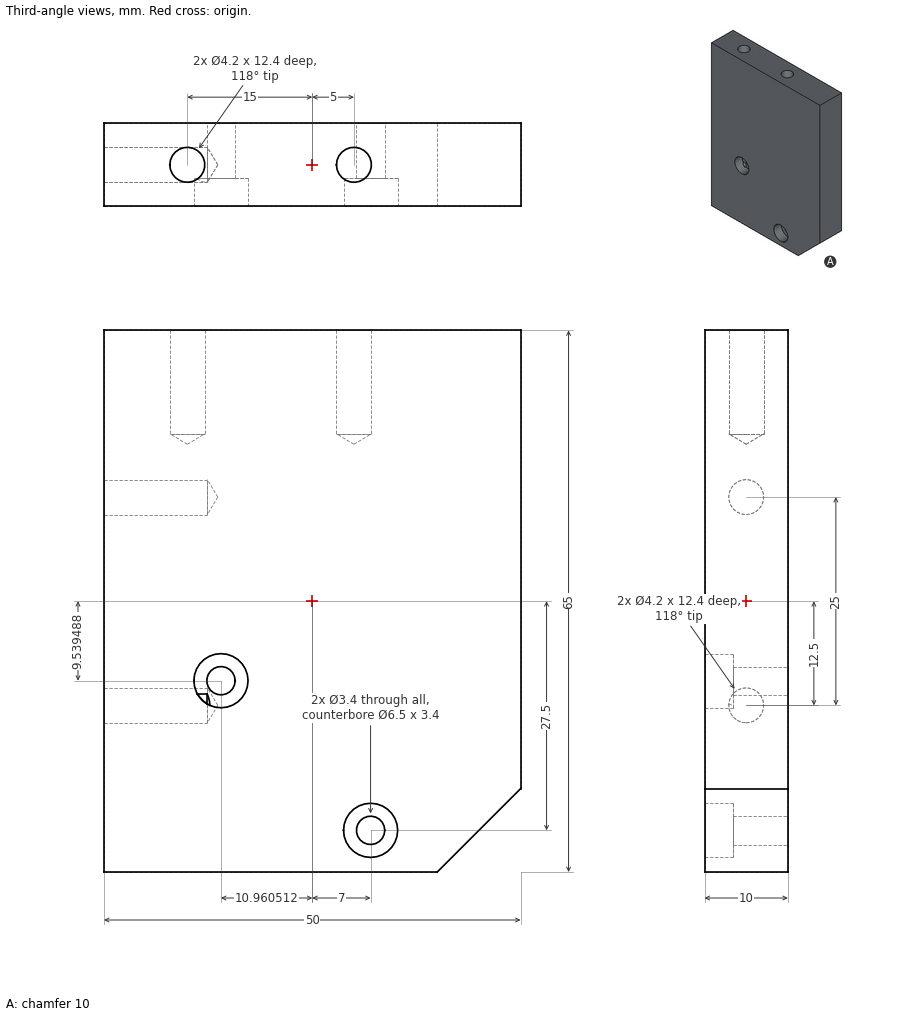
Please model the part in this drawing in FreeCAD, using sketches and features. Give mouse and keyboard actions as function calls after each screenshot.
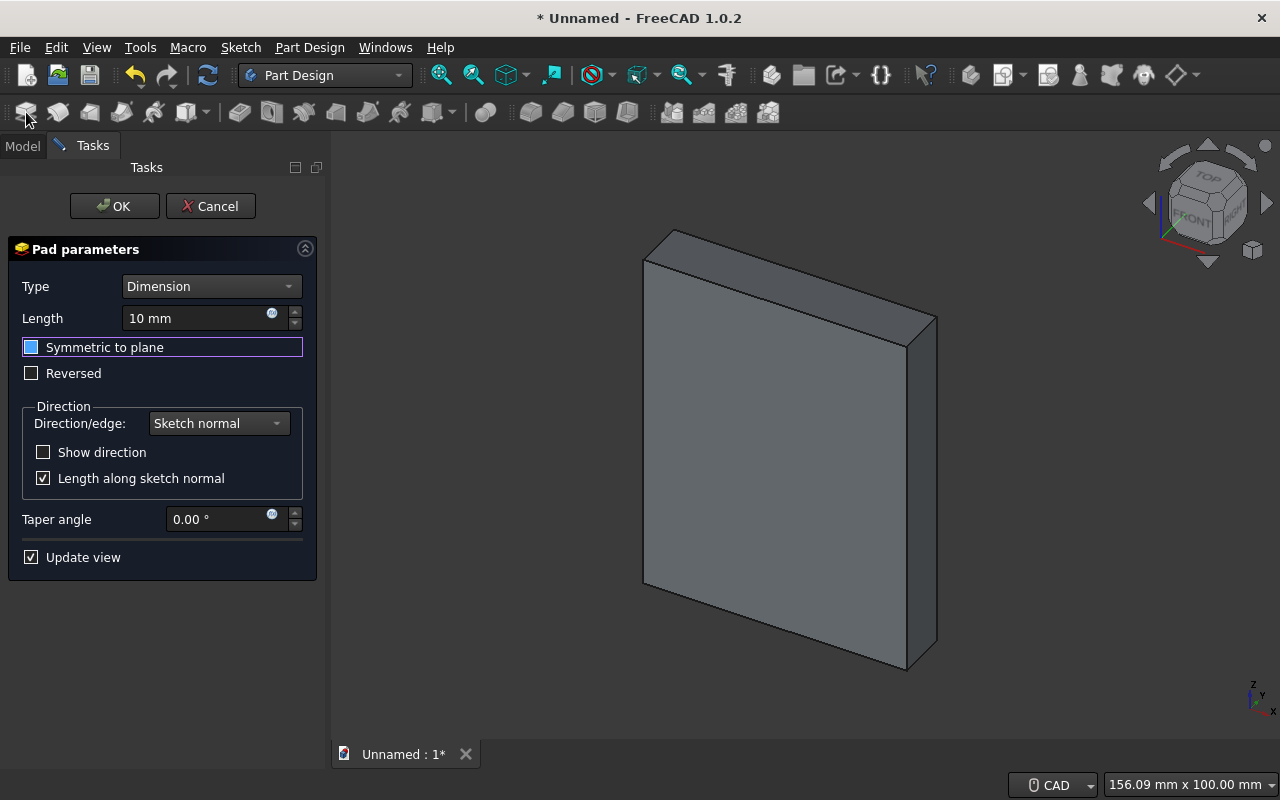
click(30, 347)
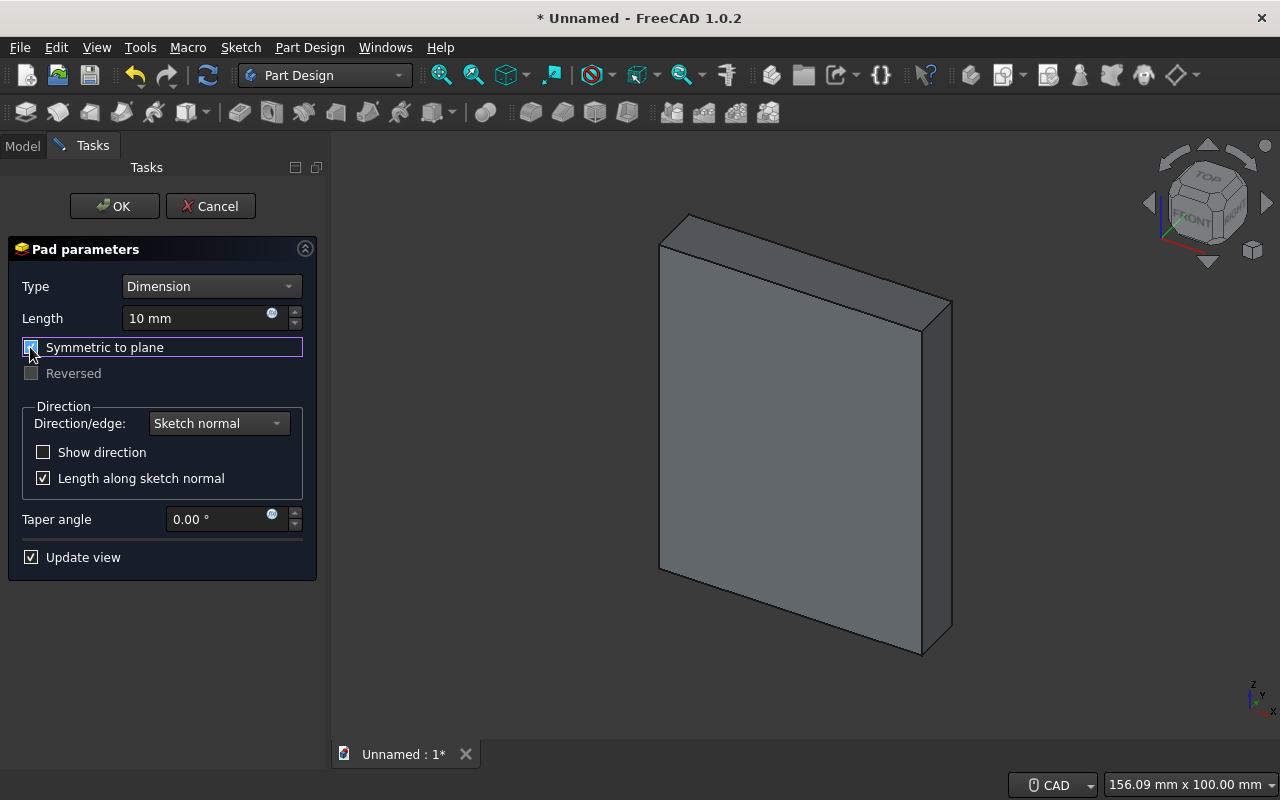
click(115, 206)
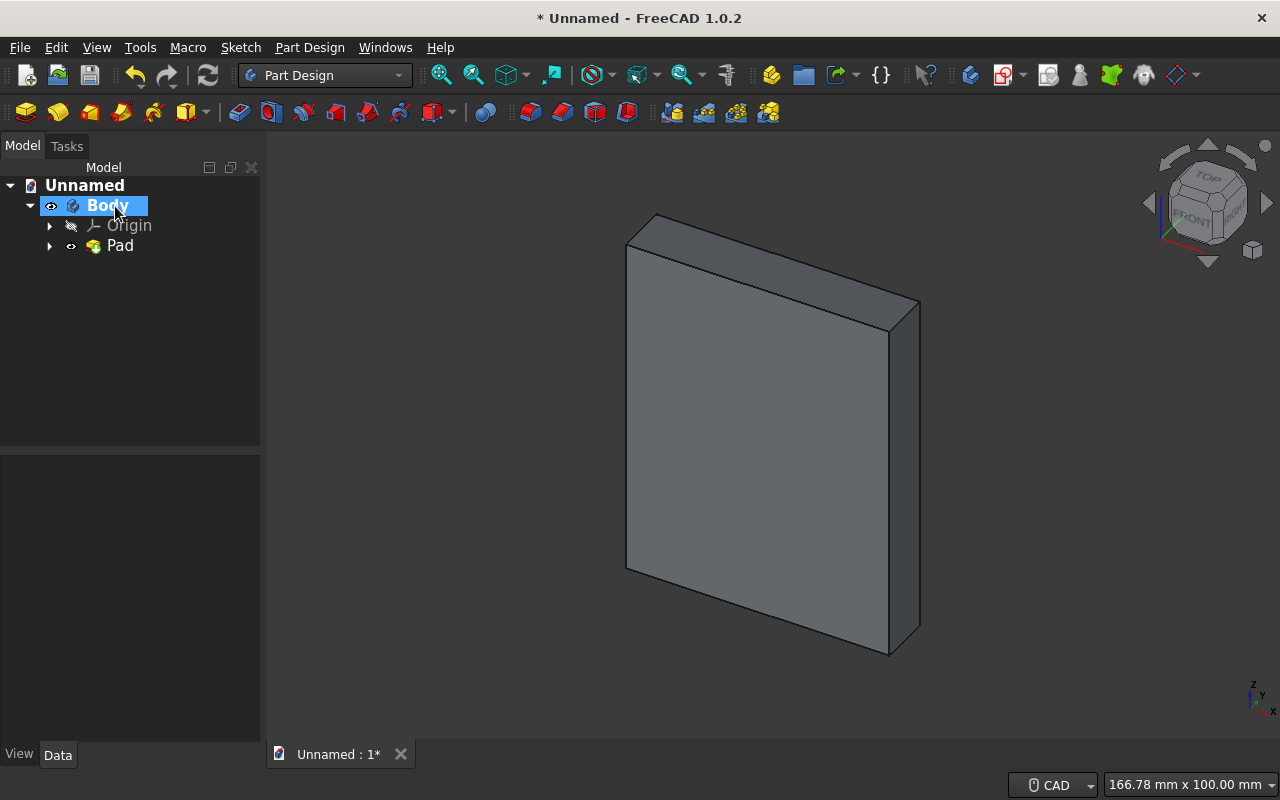
key(0)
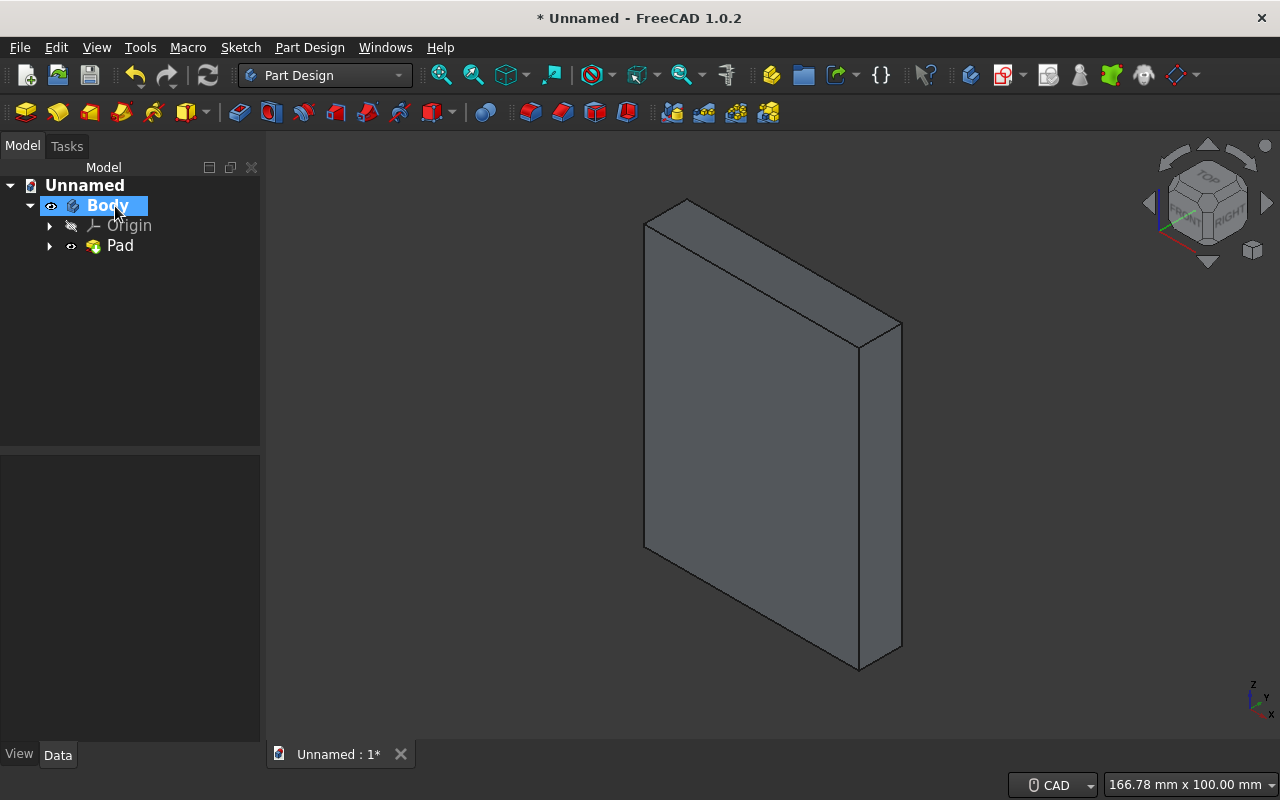
key(2)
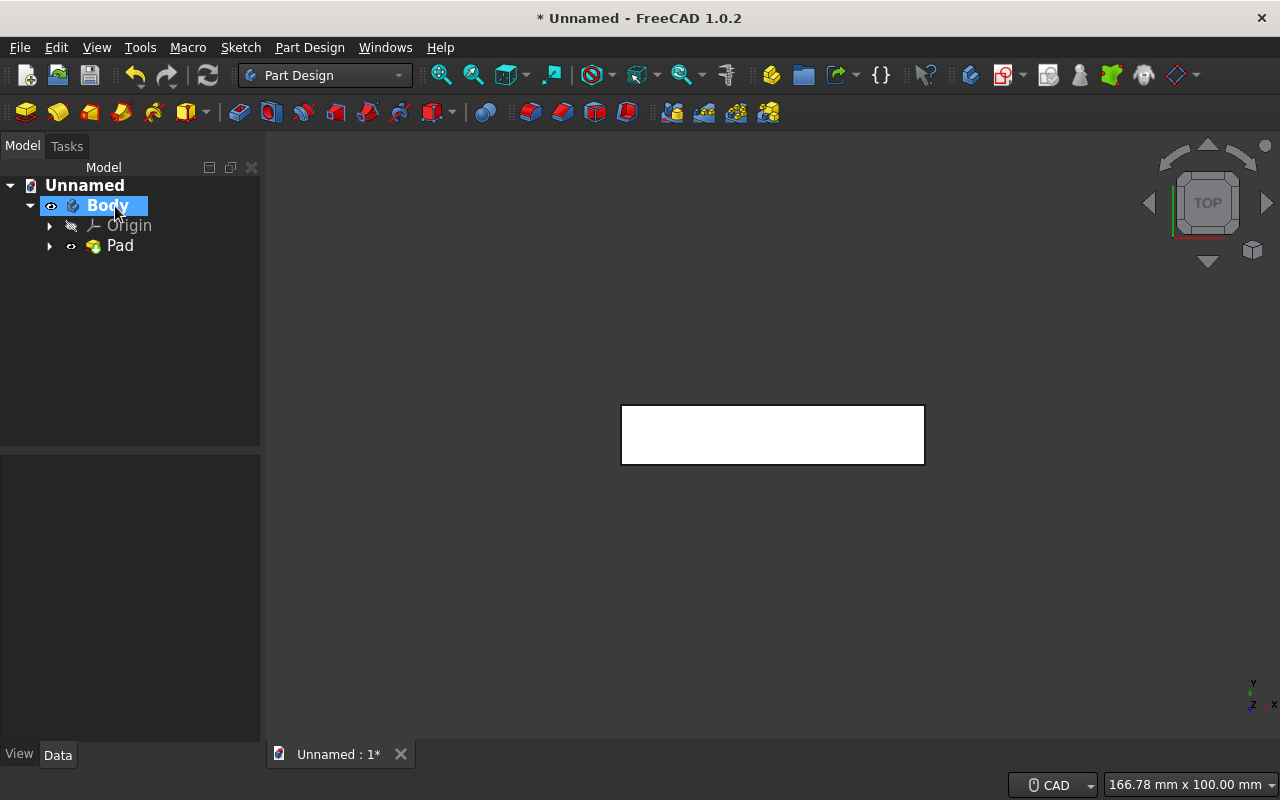
key(v)
key(f)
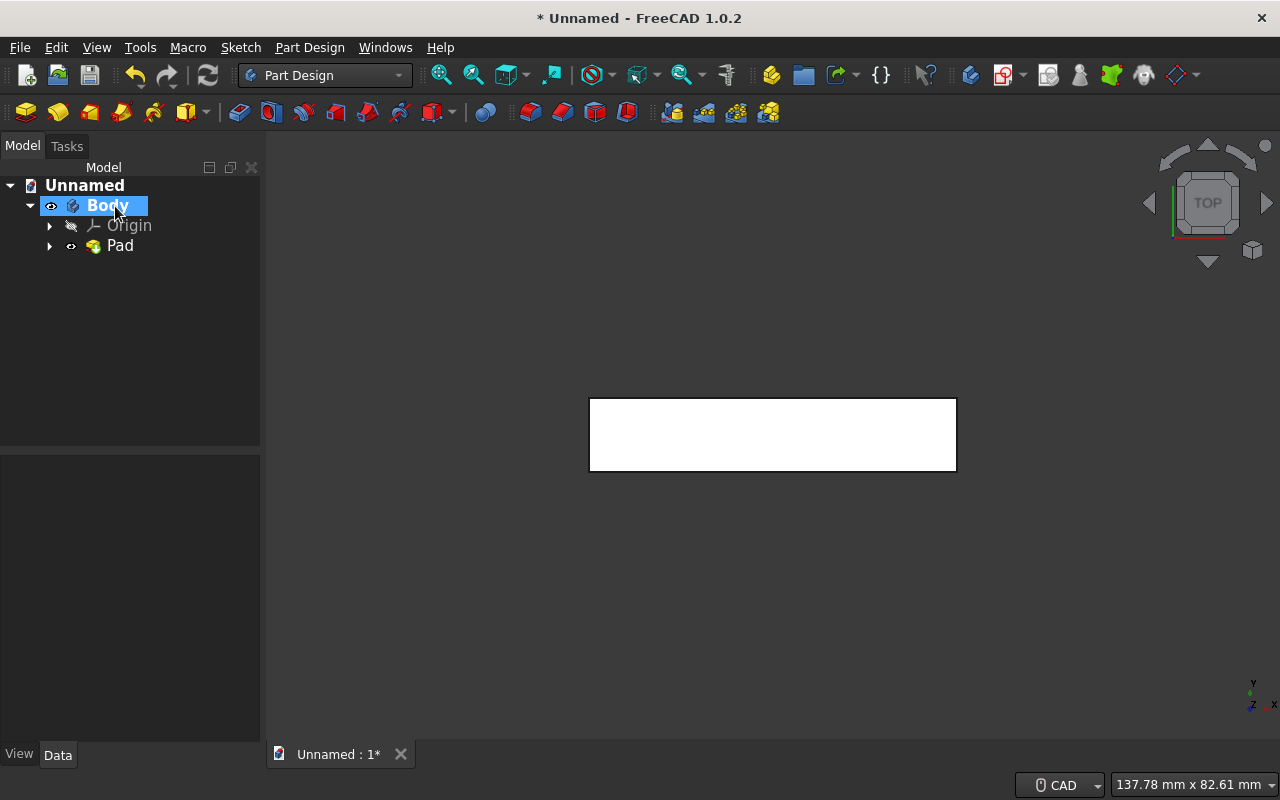
key(1)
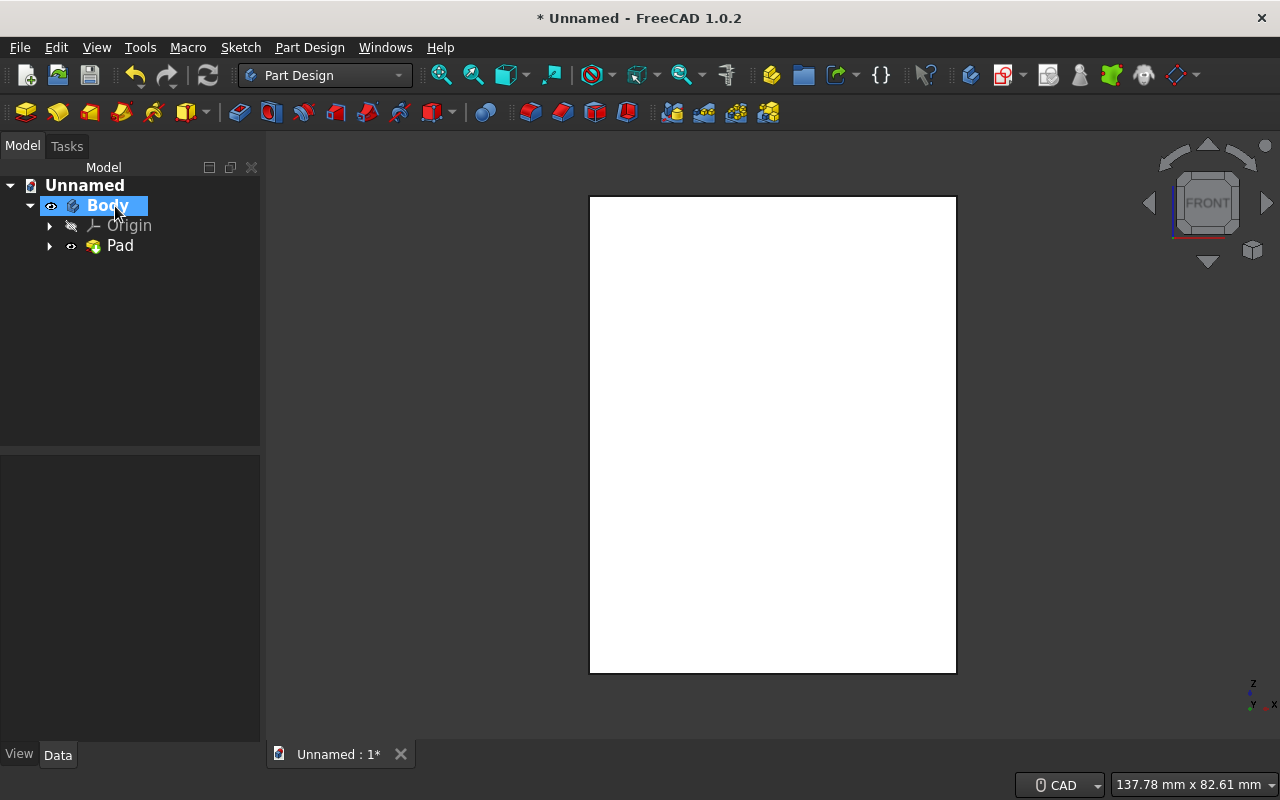
key(3)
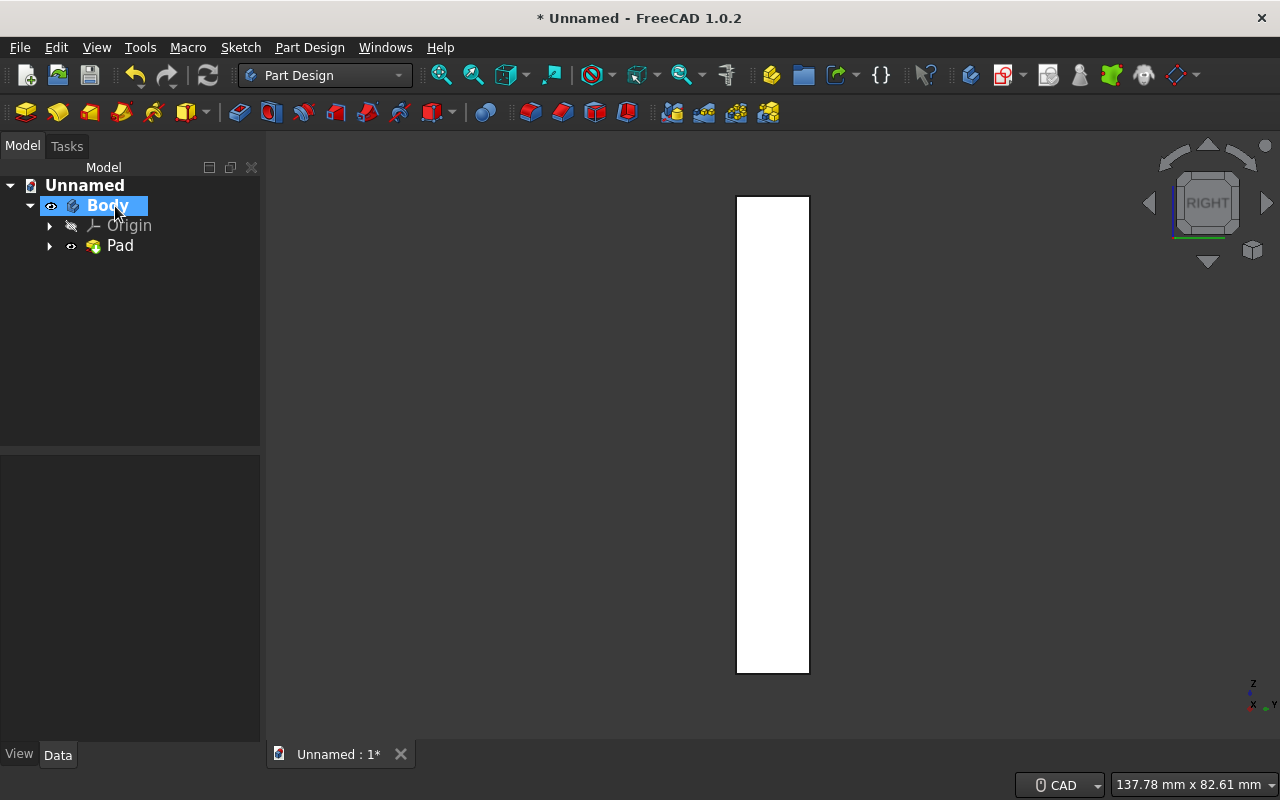
click(773, 673)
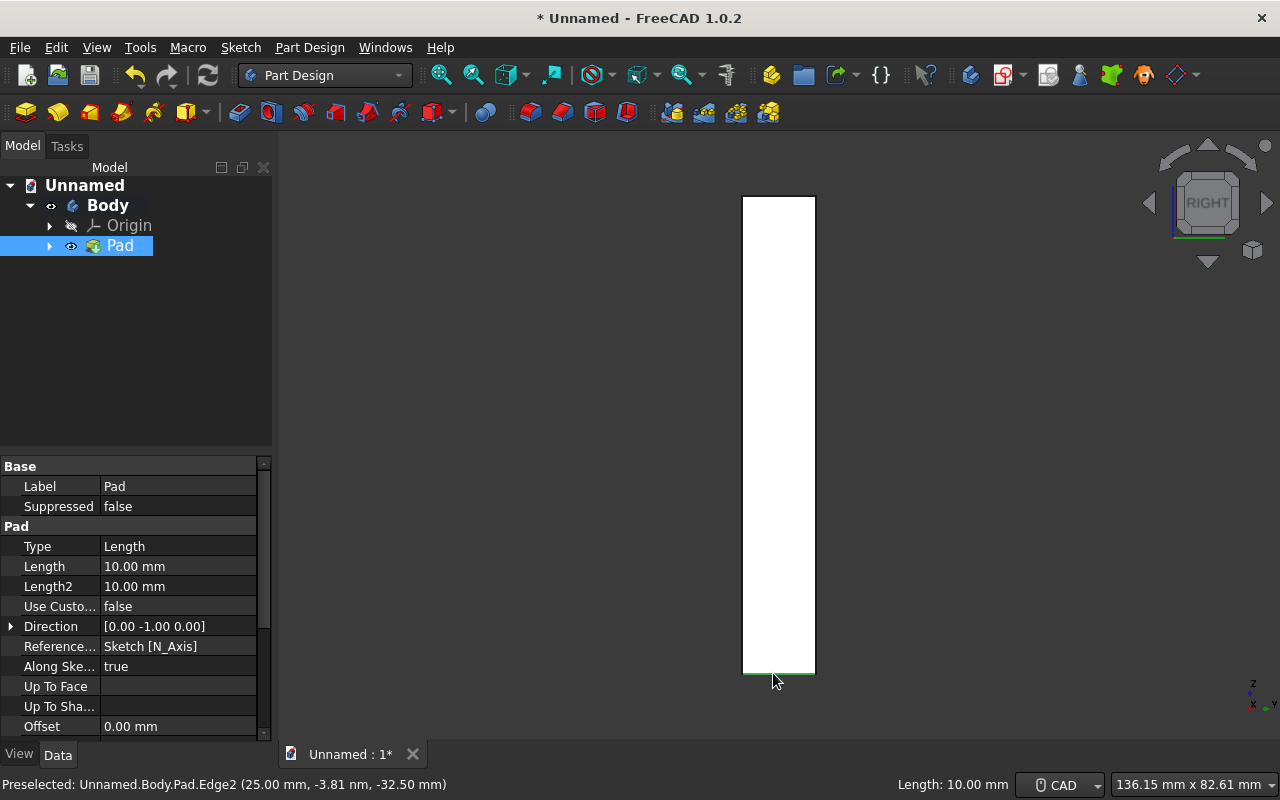
click(564, 112)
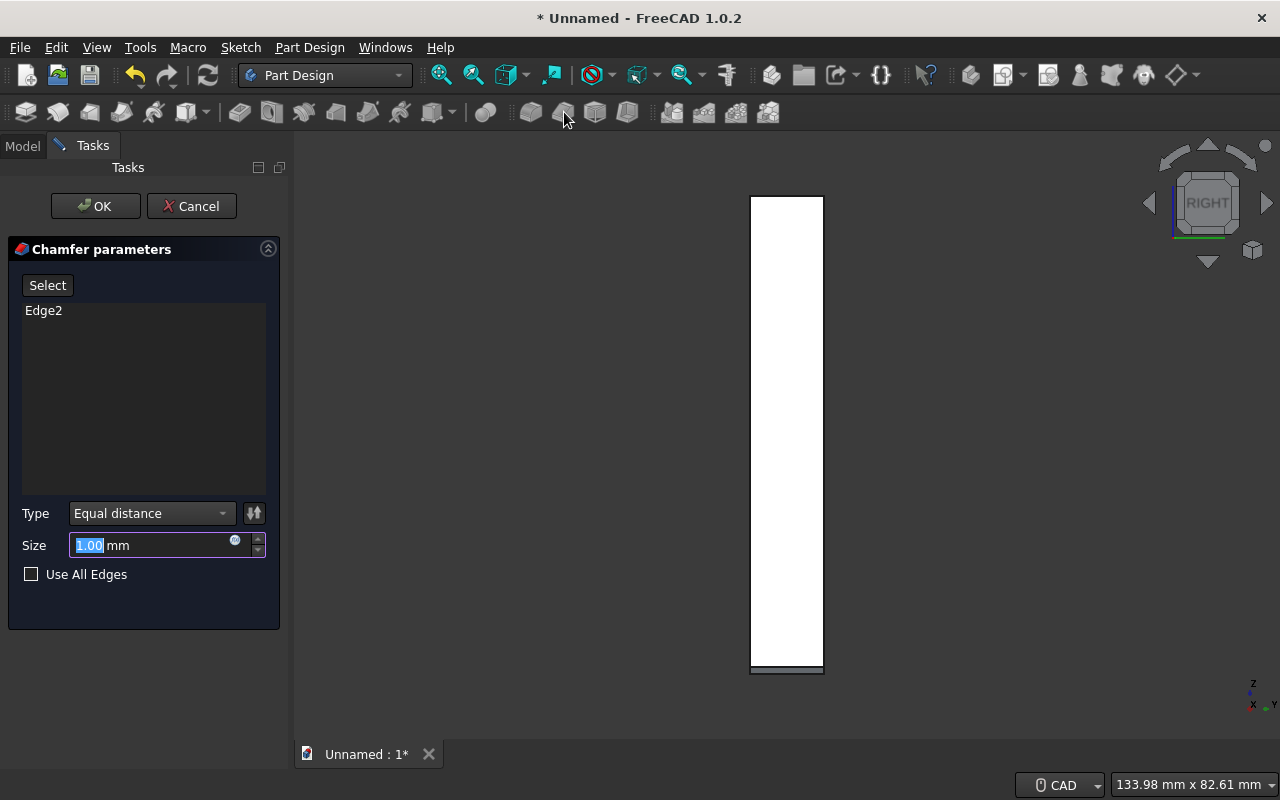
text(10)
key(Tab)